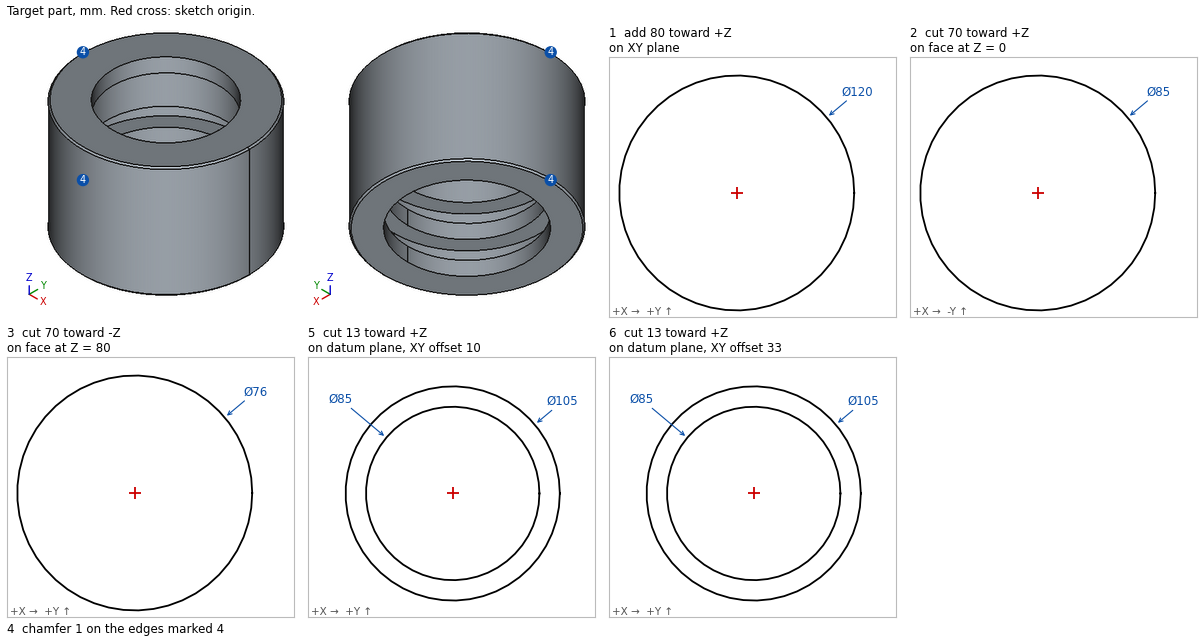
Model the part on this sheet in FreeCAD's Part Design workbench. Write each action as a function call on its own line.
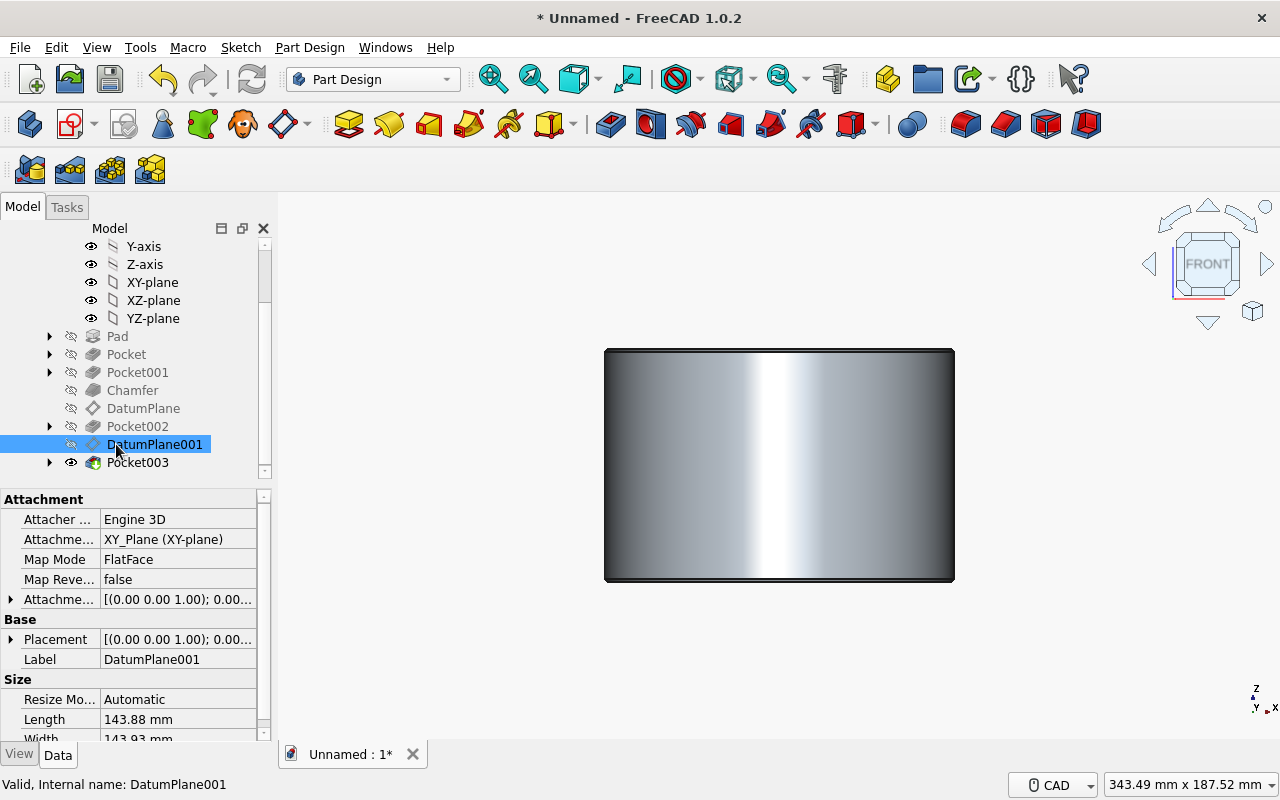
key(0)